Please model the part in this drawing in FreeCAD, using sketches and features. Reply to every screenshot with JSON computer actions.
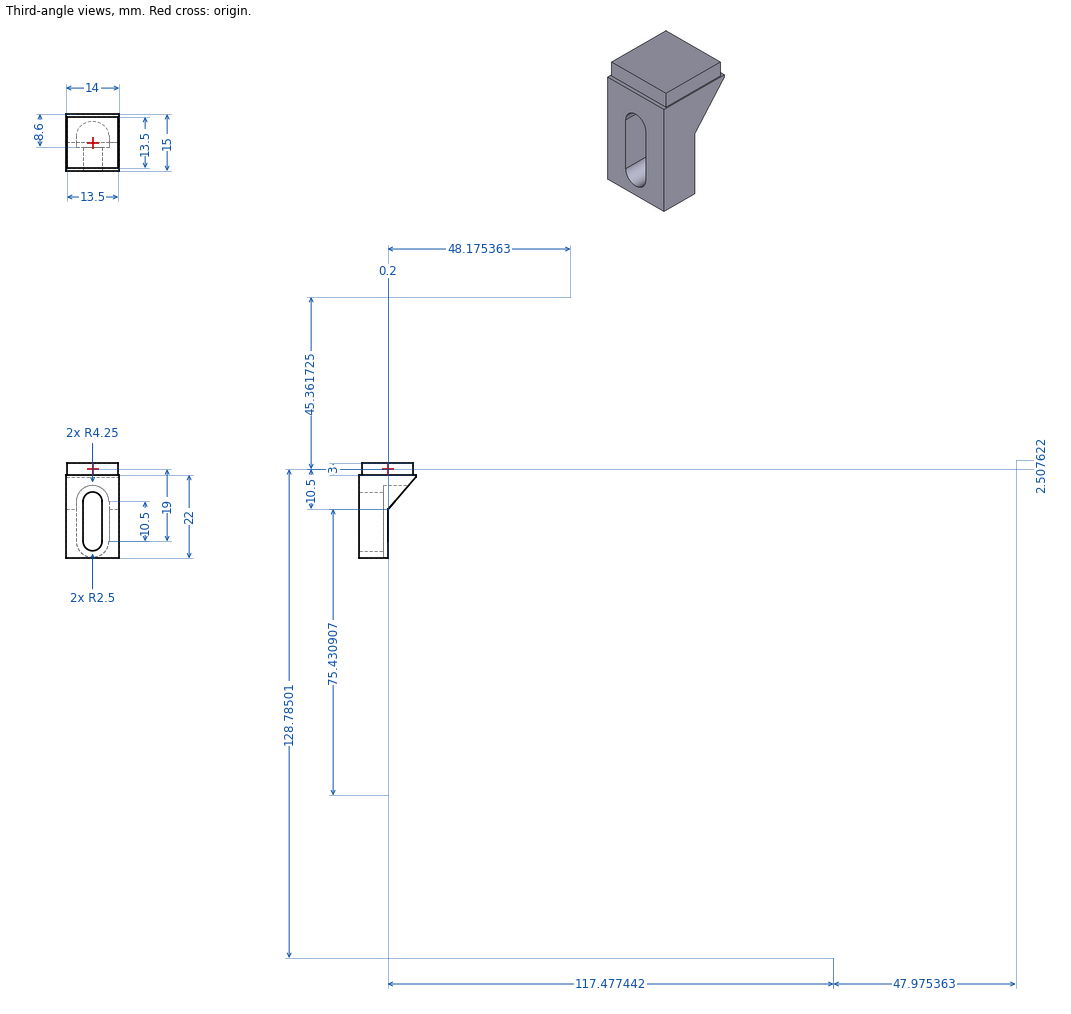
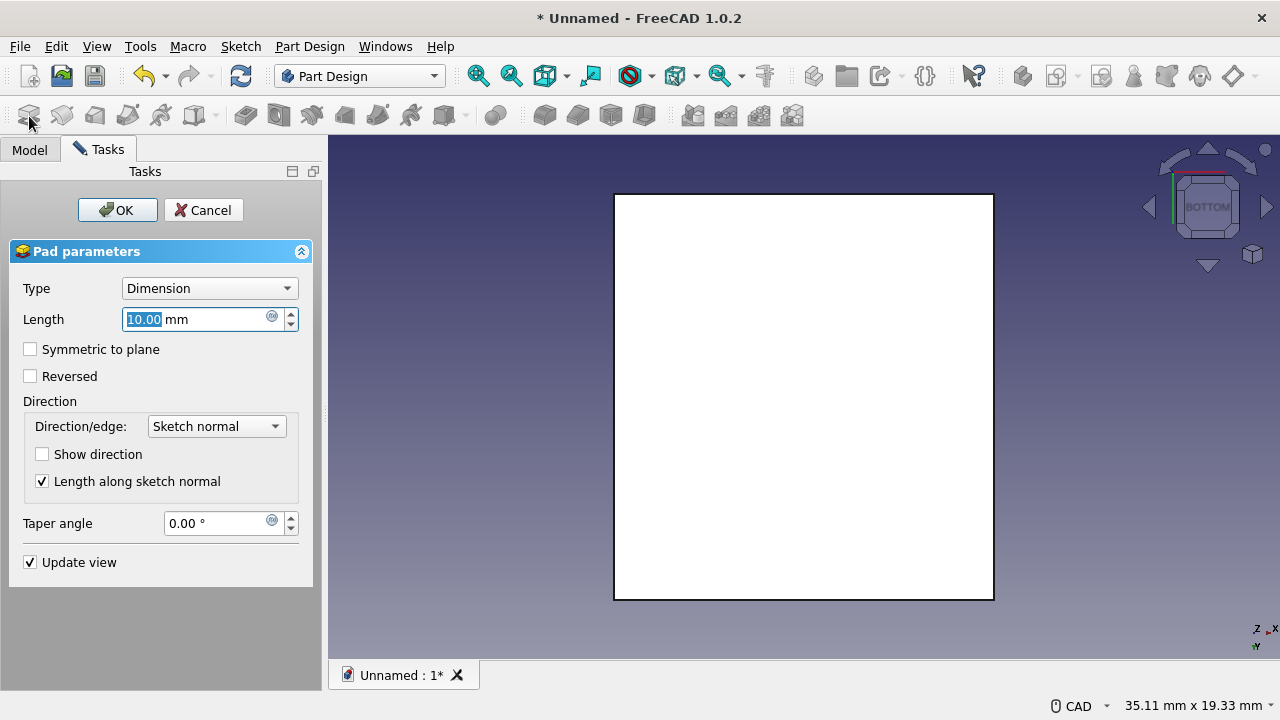
{"action": "type", "text": "22"}
{"action": "key", "text": "Tab"}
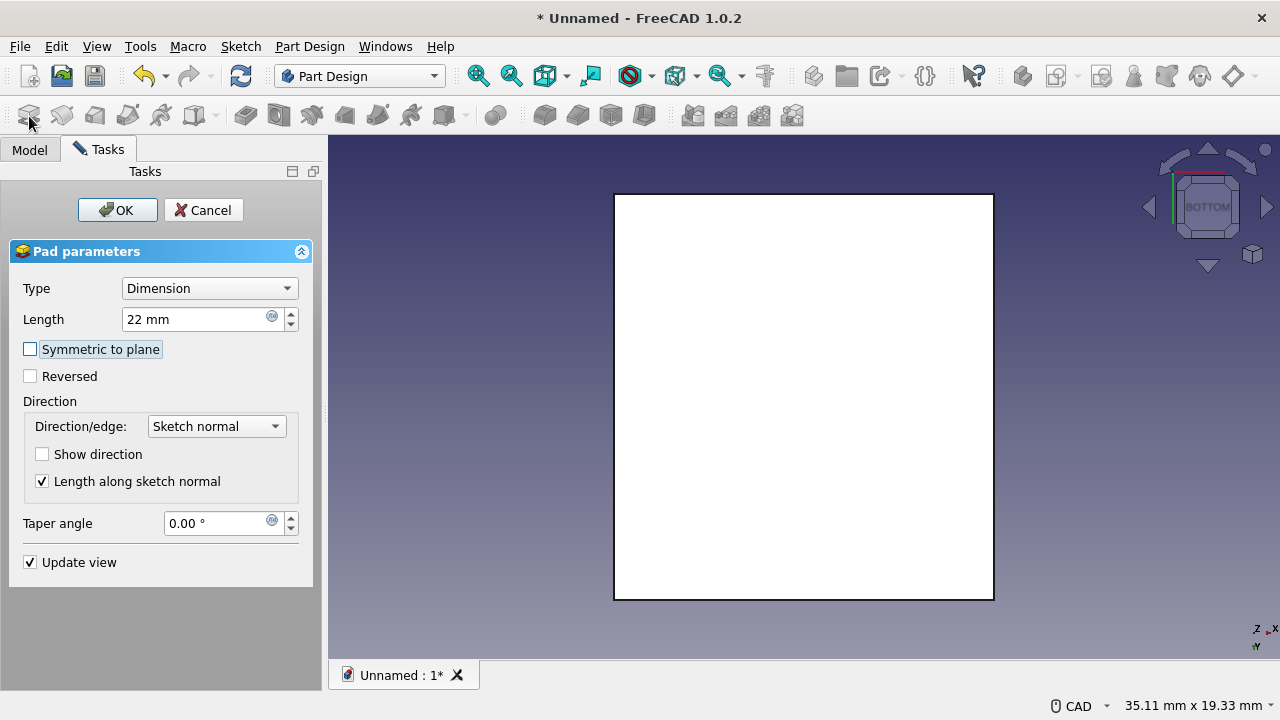
{"action": "left_click", "coordinate": [118, 210]}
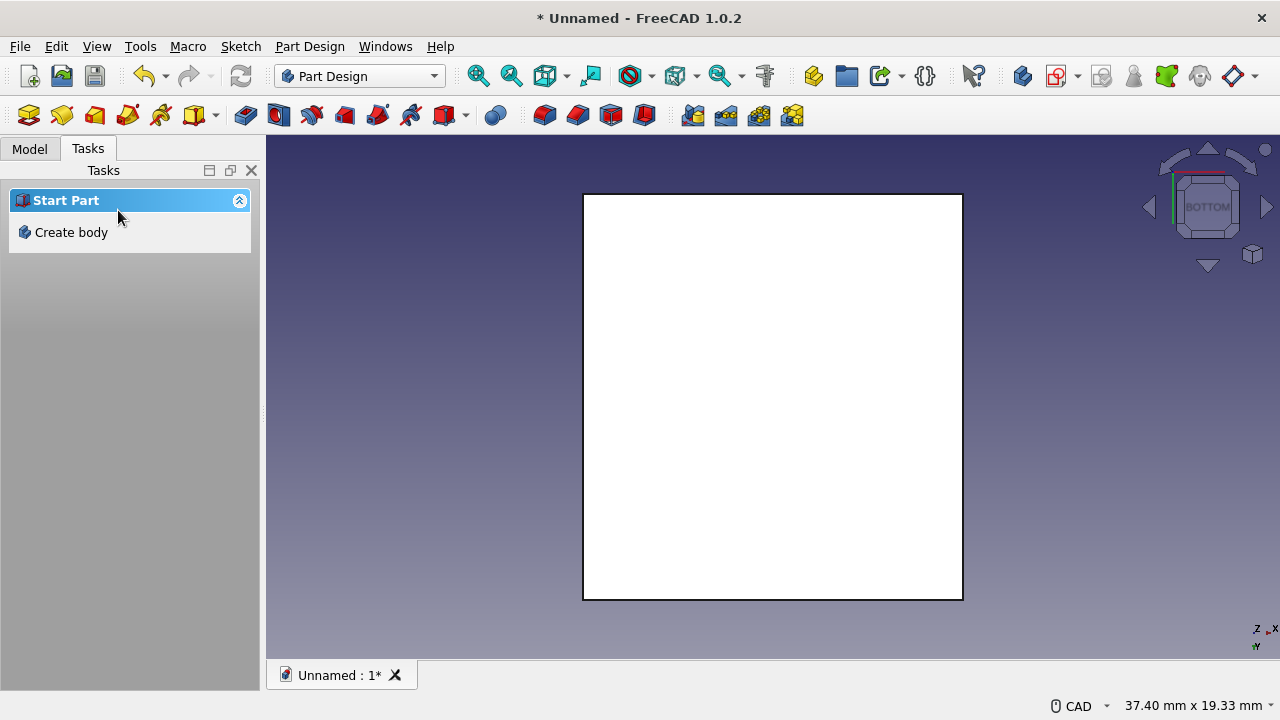
{"action": "key", "text": "0"}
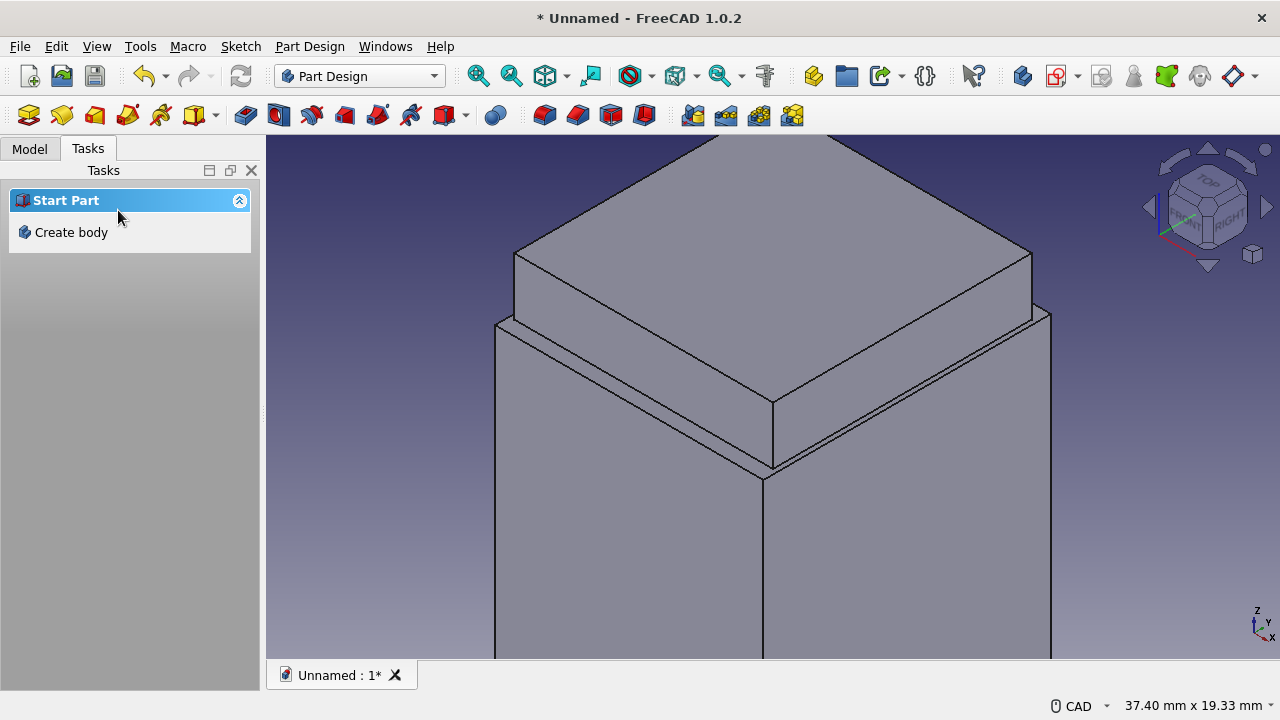
{"action": "key", "text": "v f"}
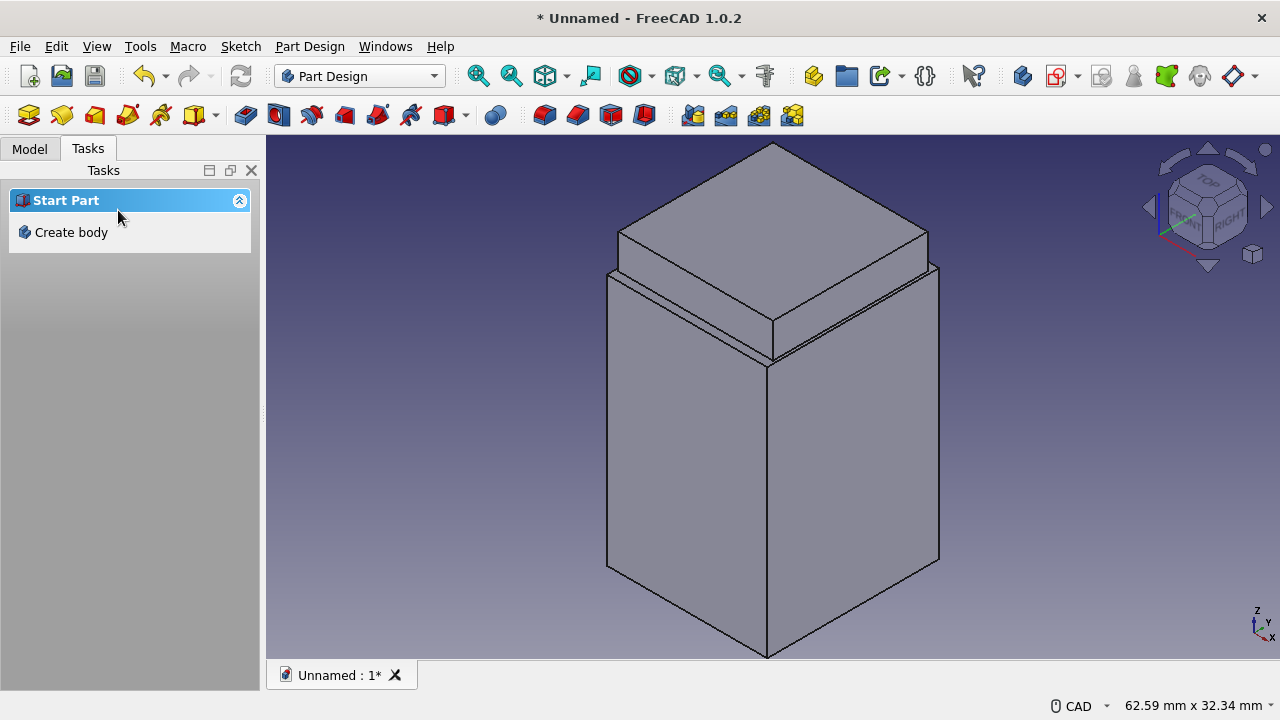
{"action": "left_click", "coordinate": [853, 421]}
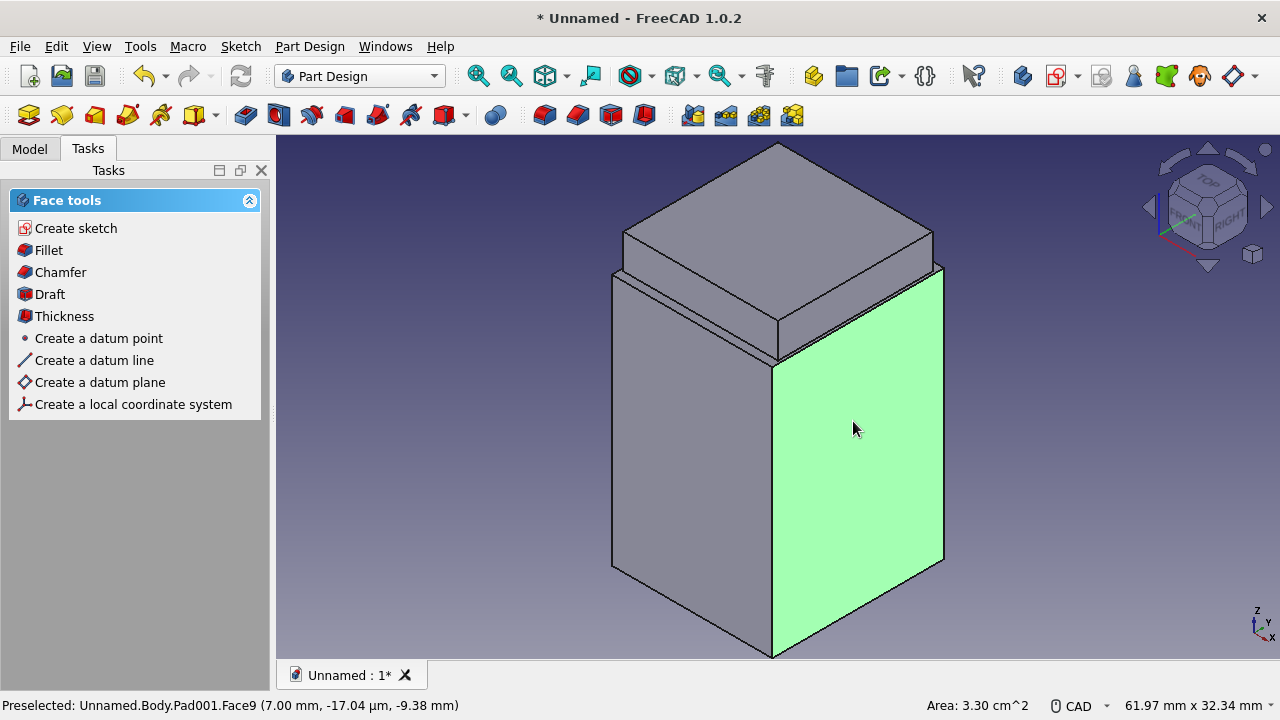
{"action": "left_click", "coordinate": [1056, 76]}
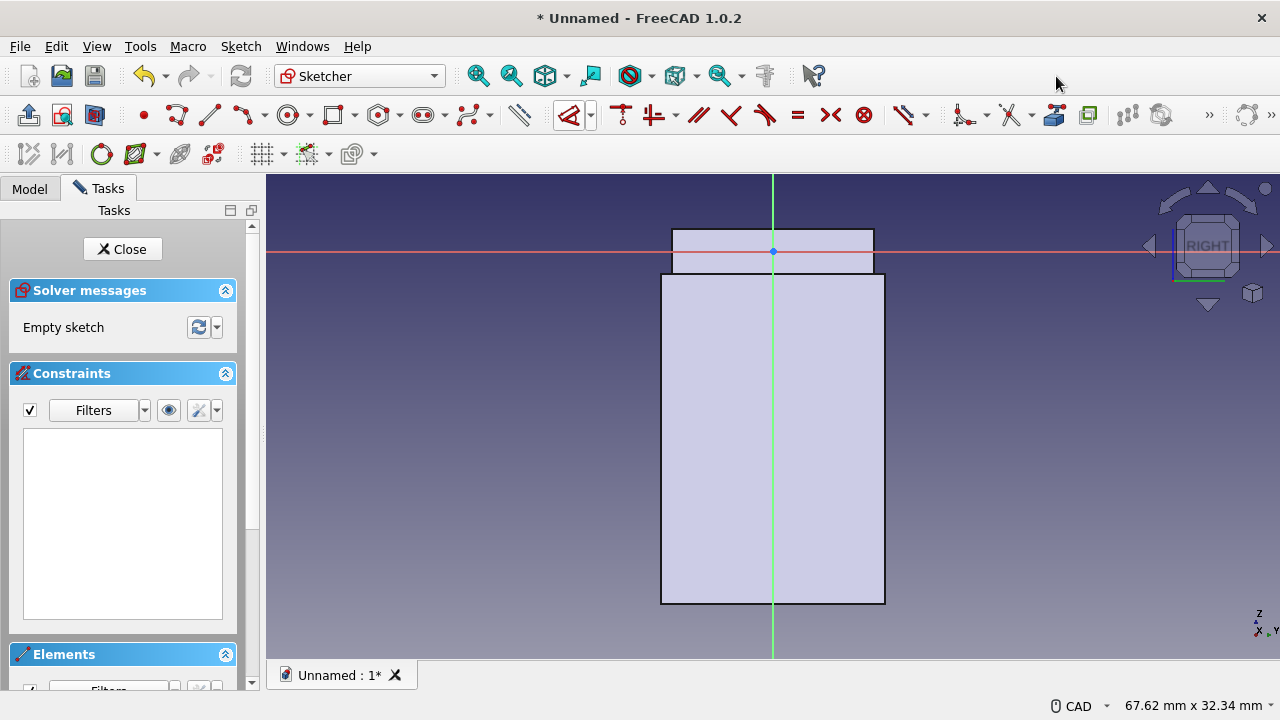
{"action": "scroll", "coordinate": [541, 359], "scroll_direction": "down", "scroll_amount": 11}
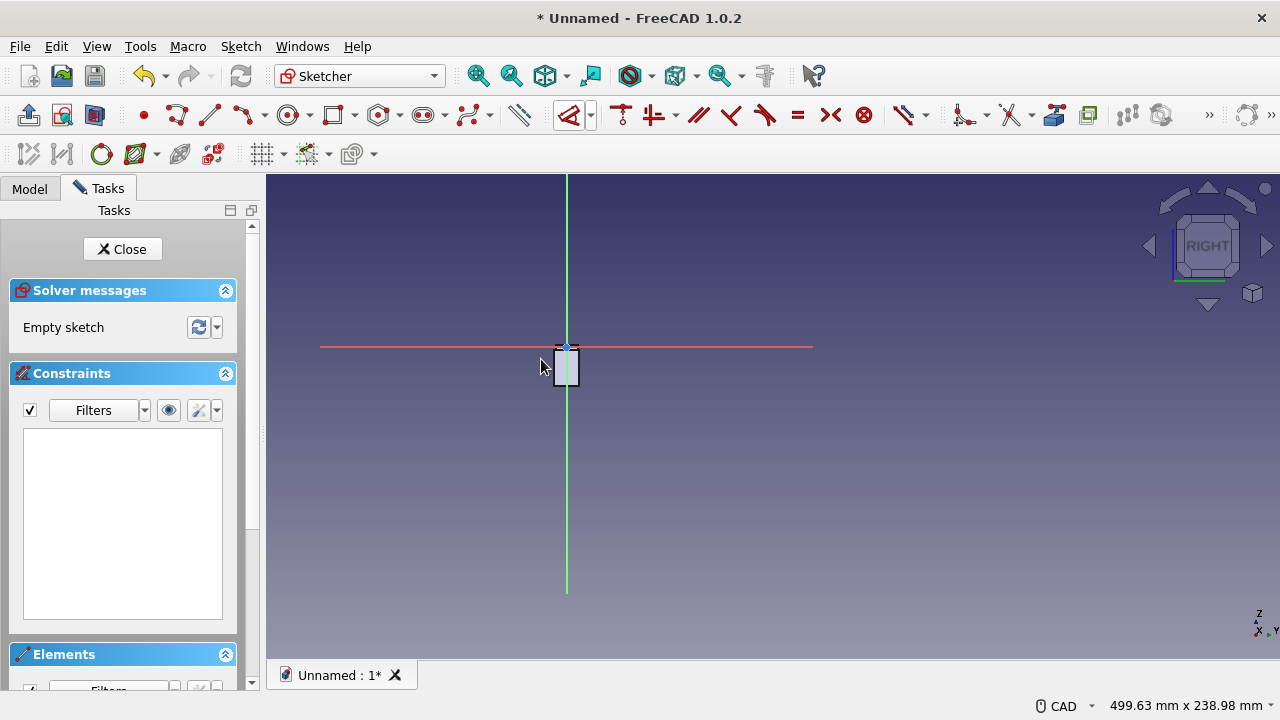
{"action": "left_click", "coordinate": [177, 116]}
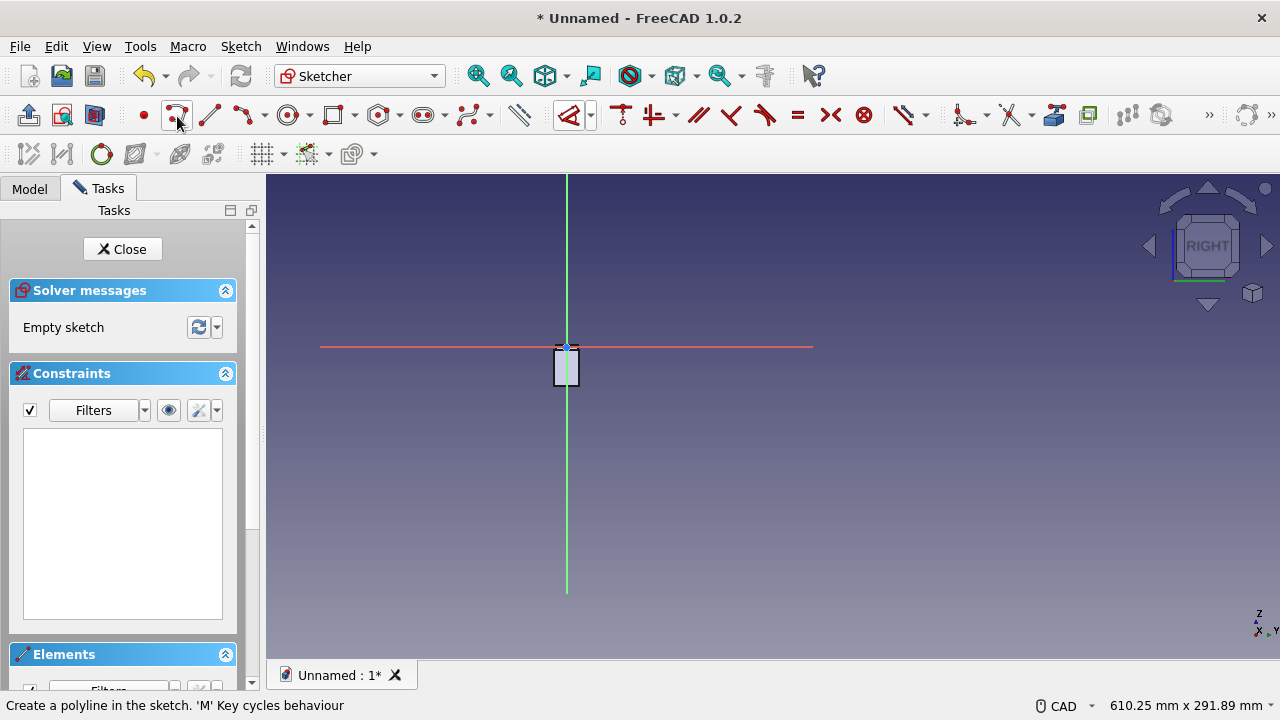
{"action": "scroll", "coordinate": [567, 365], "scroll_direction": "up", "scroll_amount": 20}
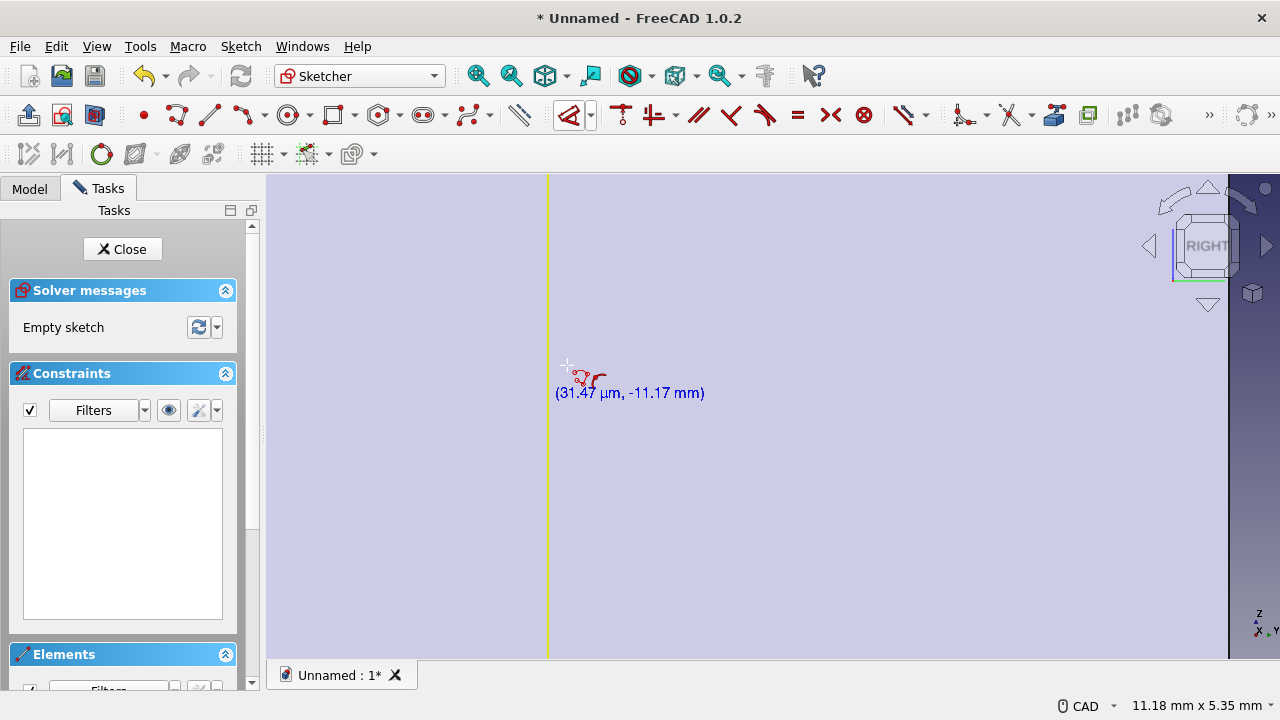
{"action": "left_click", "coordinate": [566, 337]}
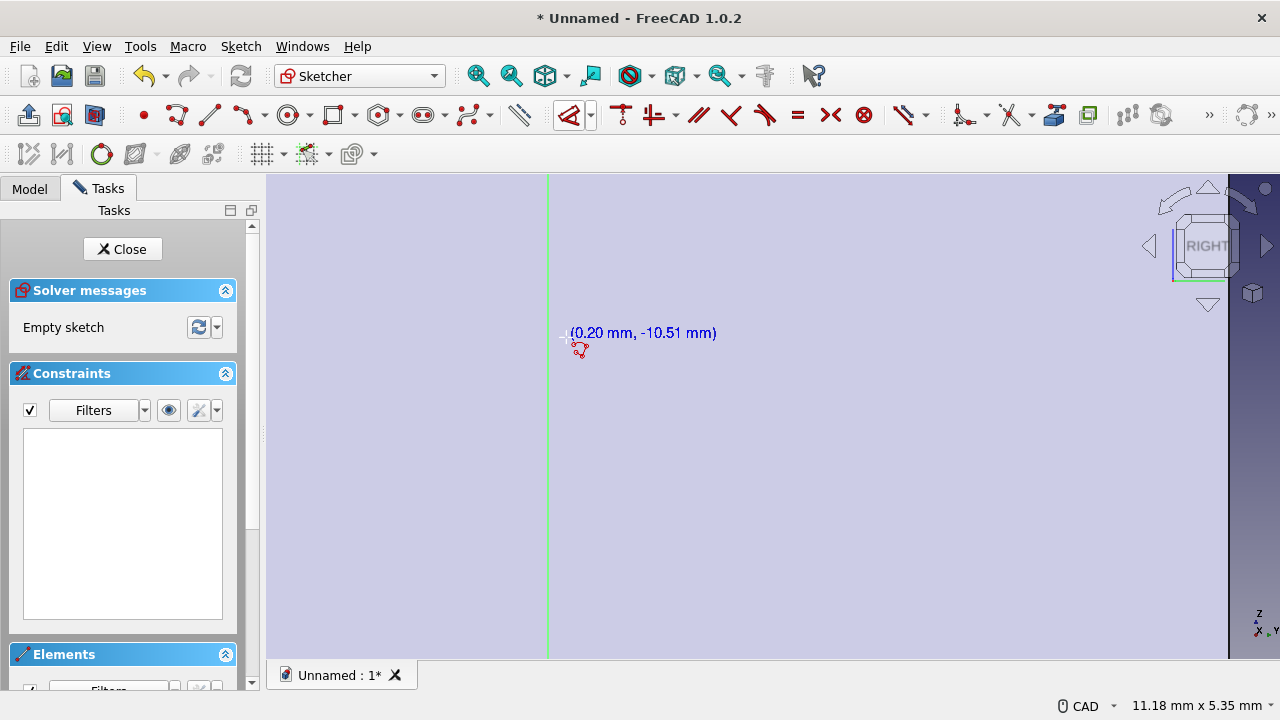
{"action": "scroll", "coordinate": [704, 416], "scroll_direction": "down", "scroll_amount": 15}